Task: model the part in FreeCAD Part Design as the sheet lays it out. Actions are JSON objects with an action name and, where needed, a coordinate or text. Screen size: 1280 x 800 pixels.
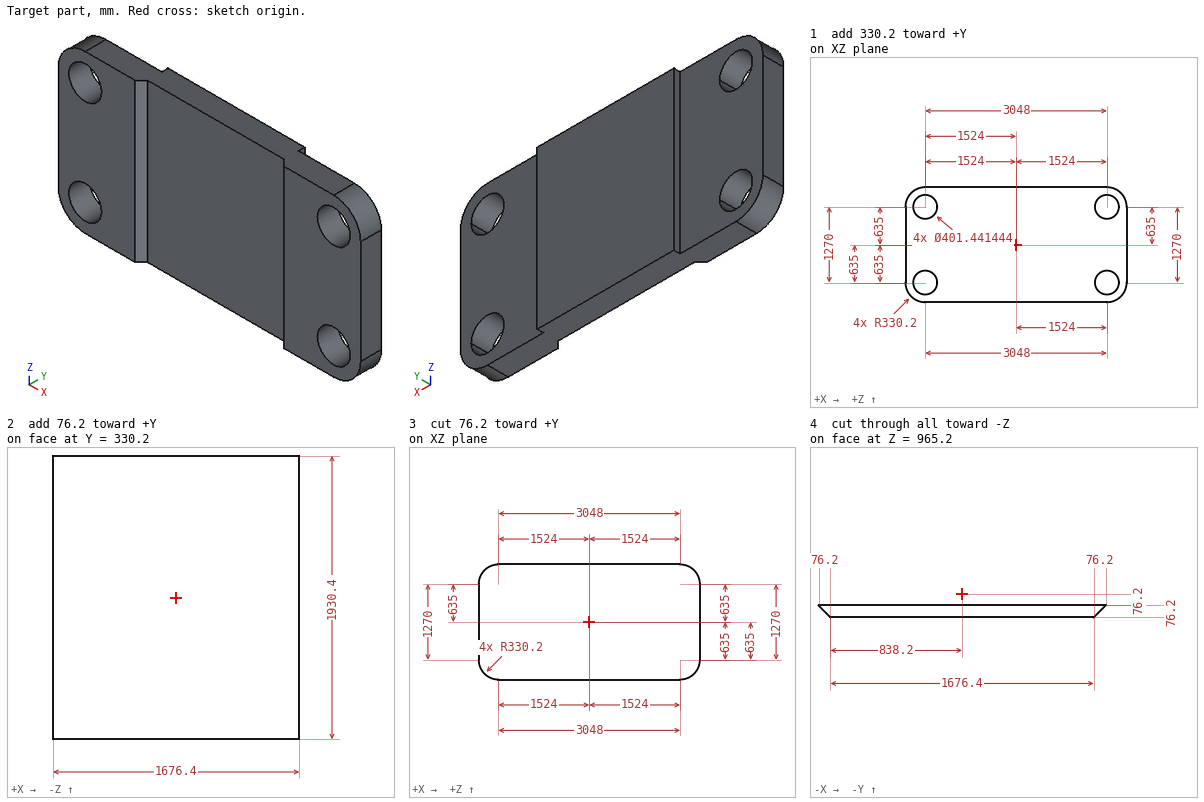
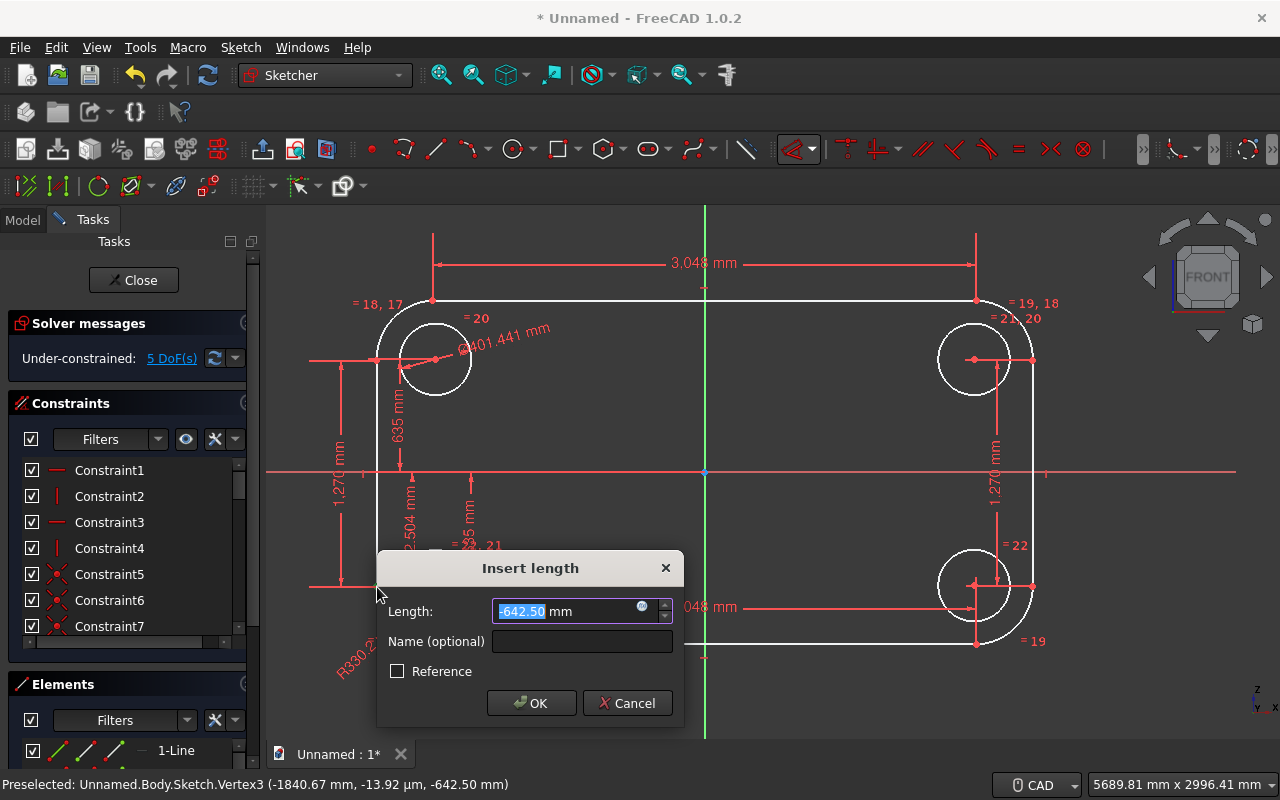
{"action": "type", "text": "-635"}
{"action": "key", "text": "Return"}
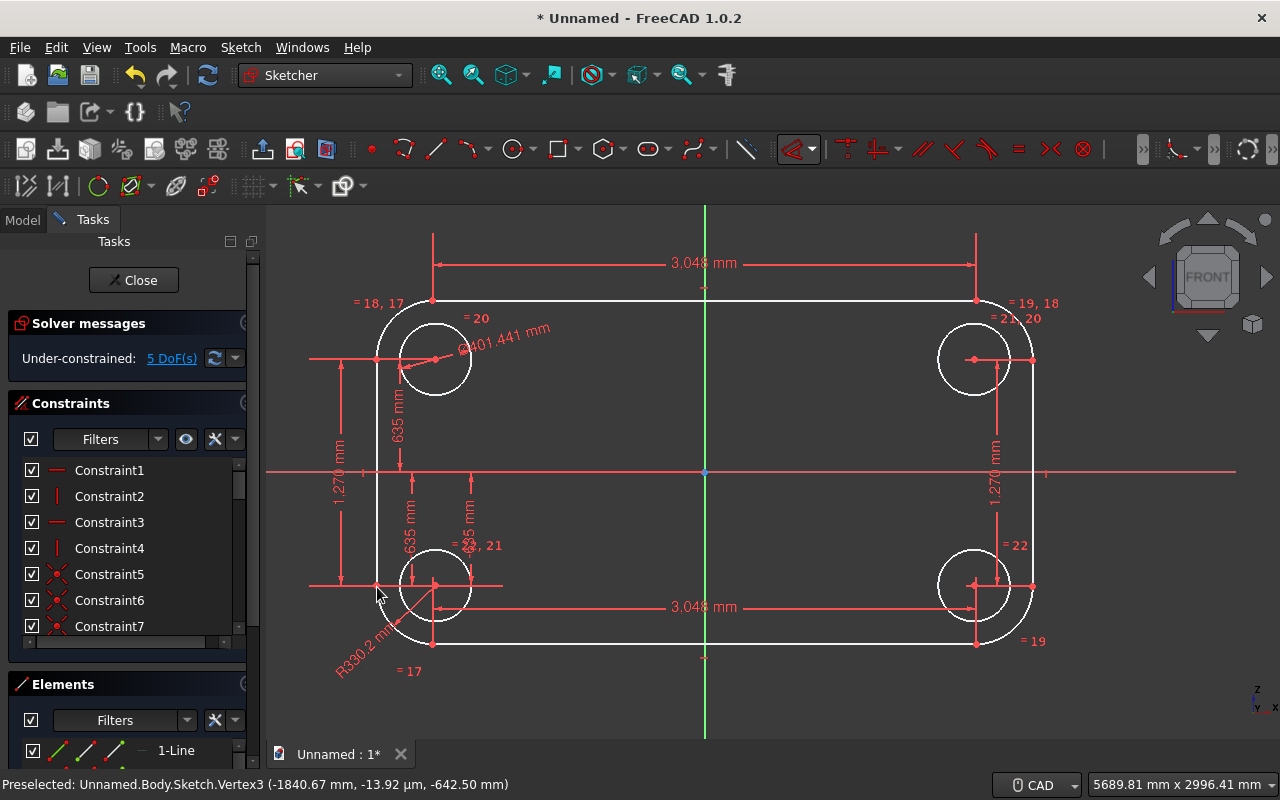
{"action": "left_click", "coordinate": [1033, 360]}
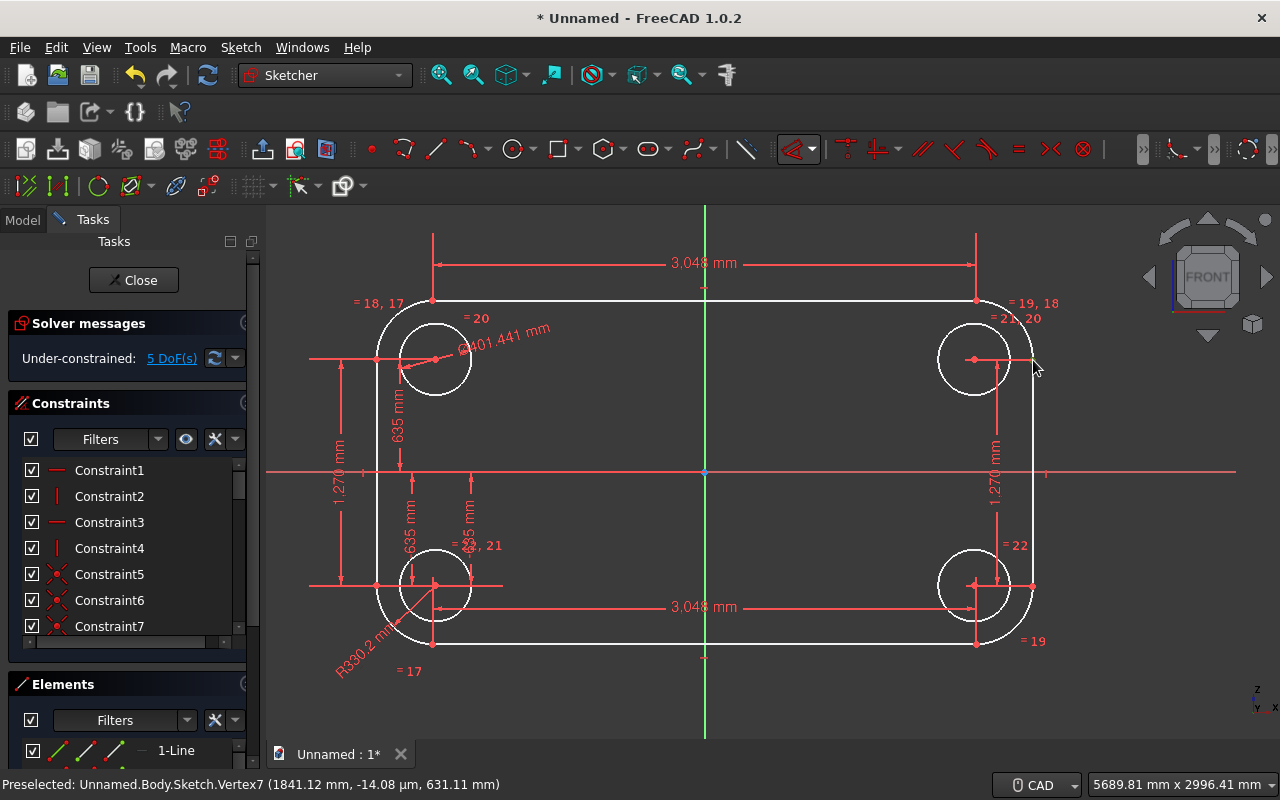
{"action": "left_click", "coordinate": [814, 150]}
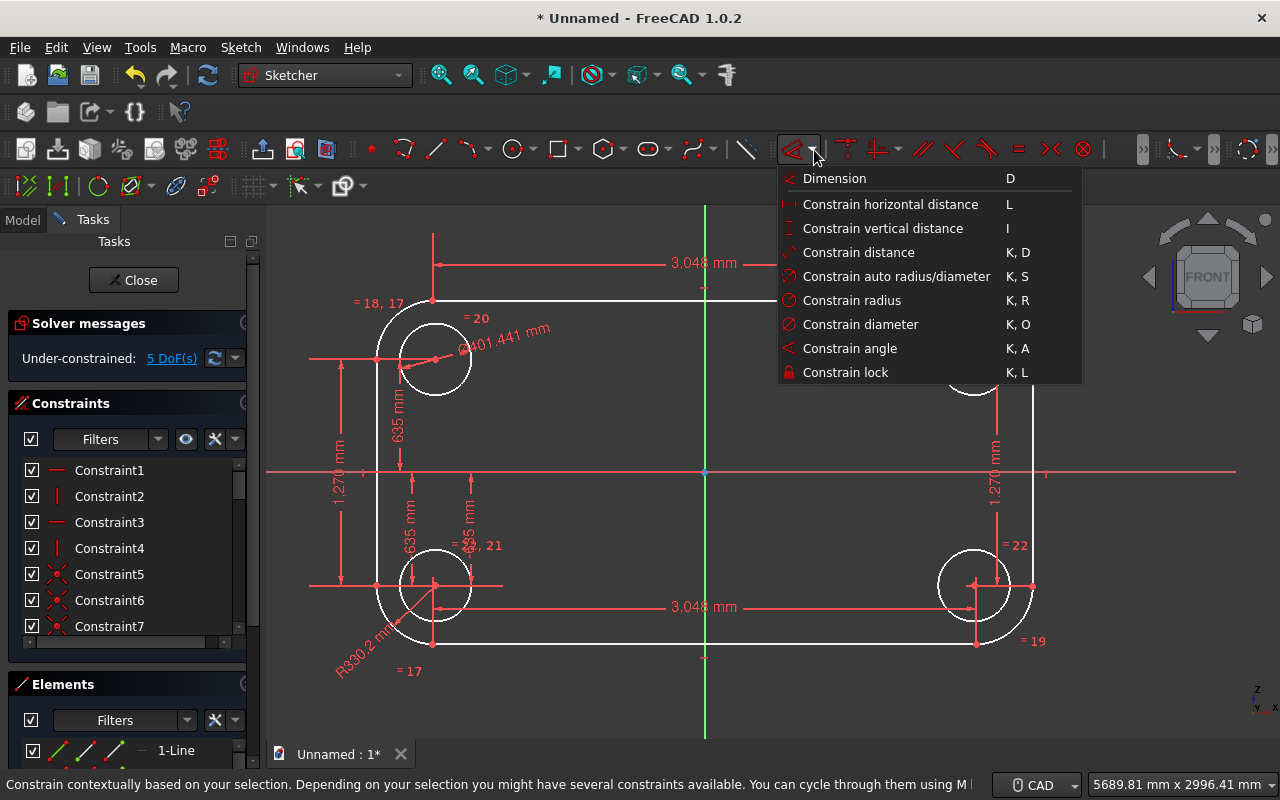
{"action": "left_click", "coordinate": [930, 228]}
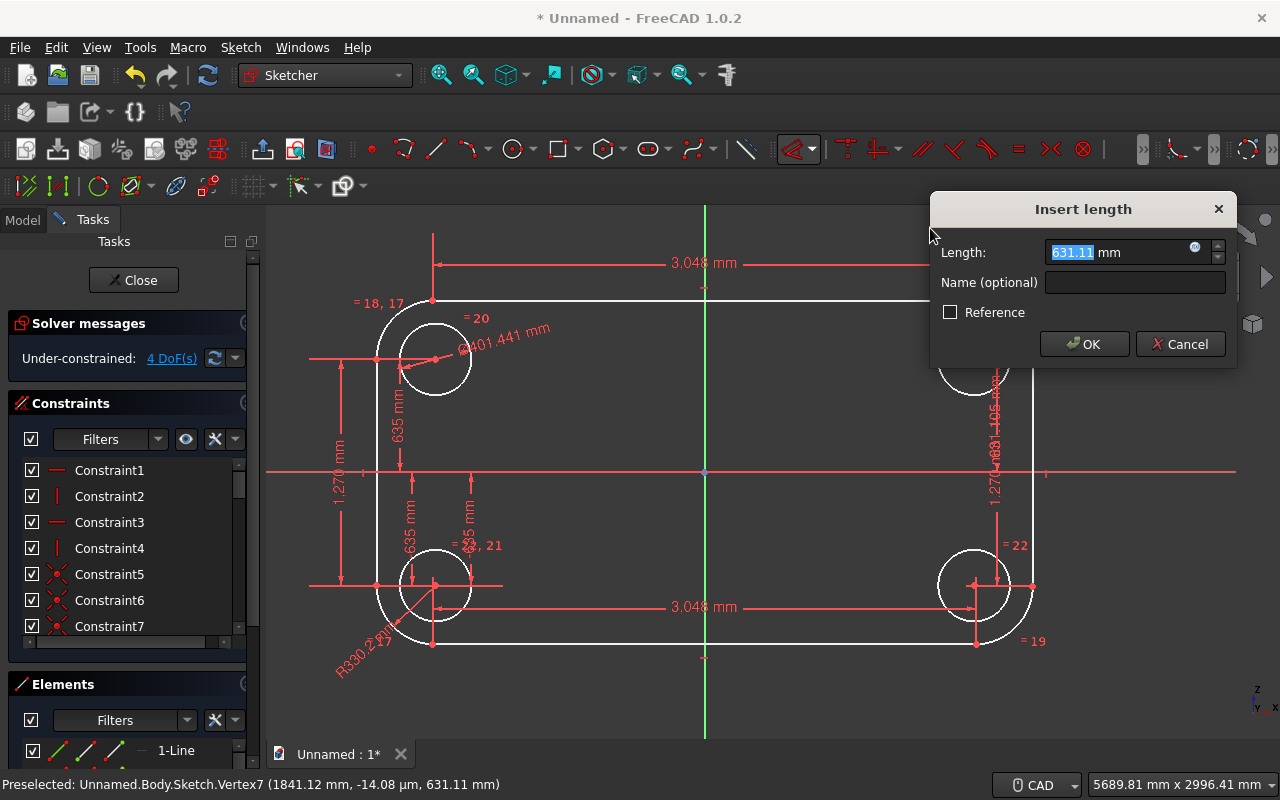
{"action": "type", "text": "635"}
{"action": "key", "text": "Return"}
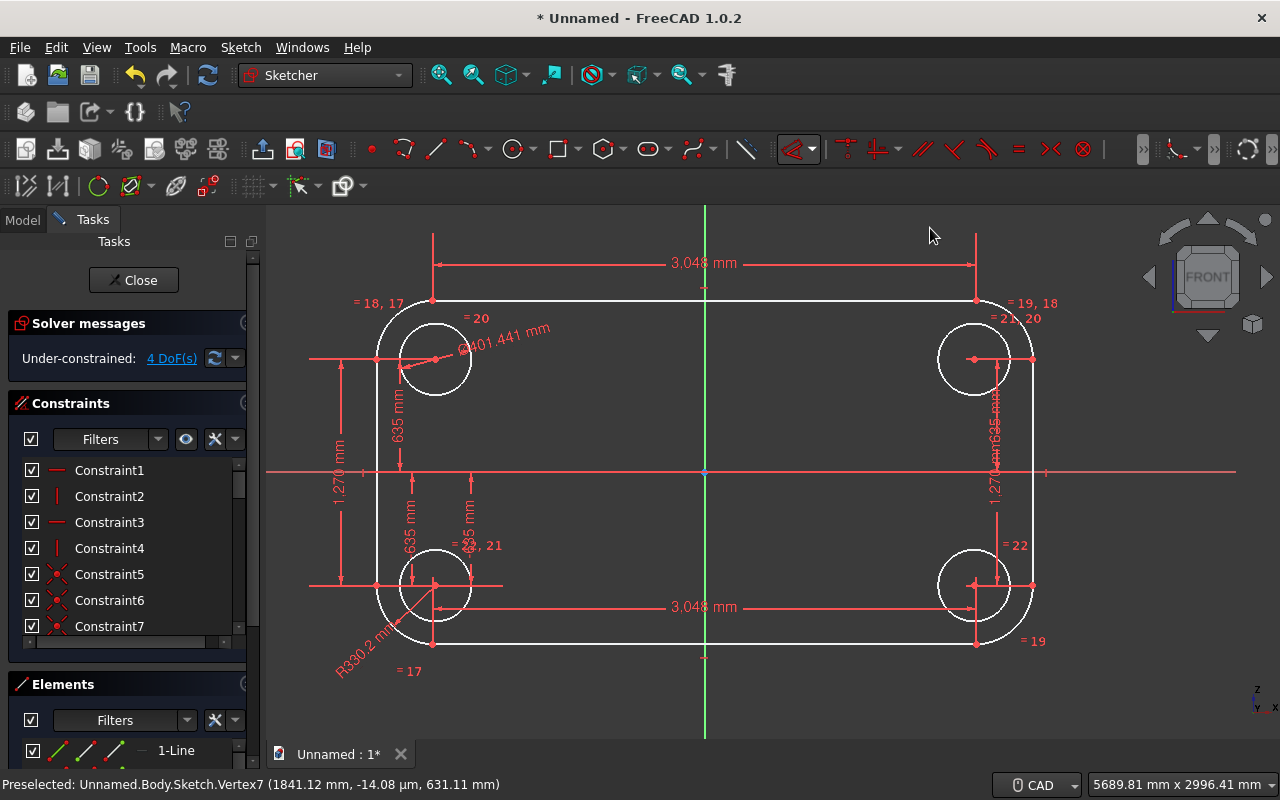
{"action": "left_click", "coordinate": [436, 359]}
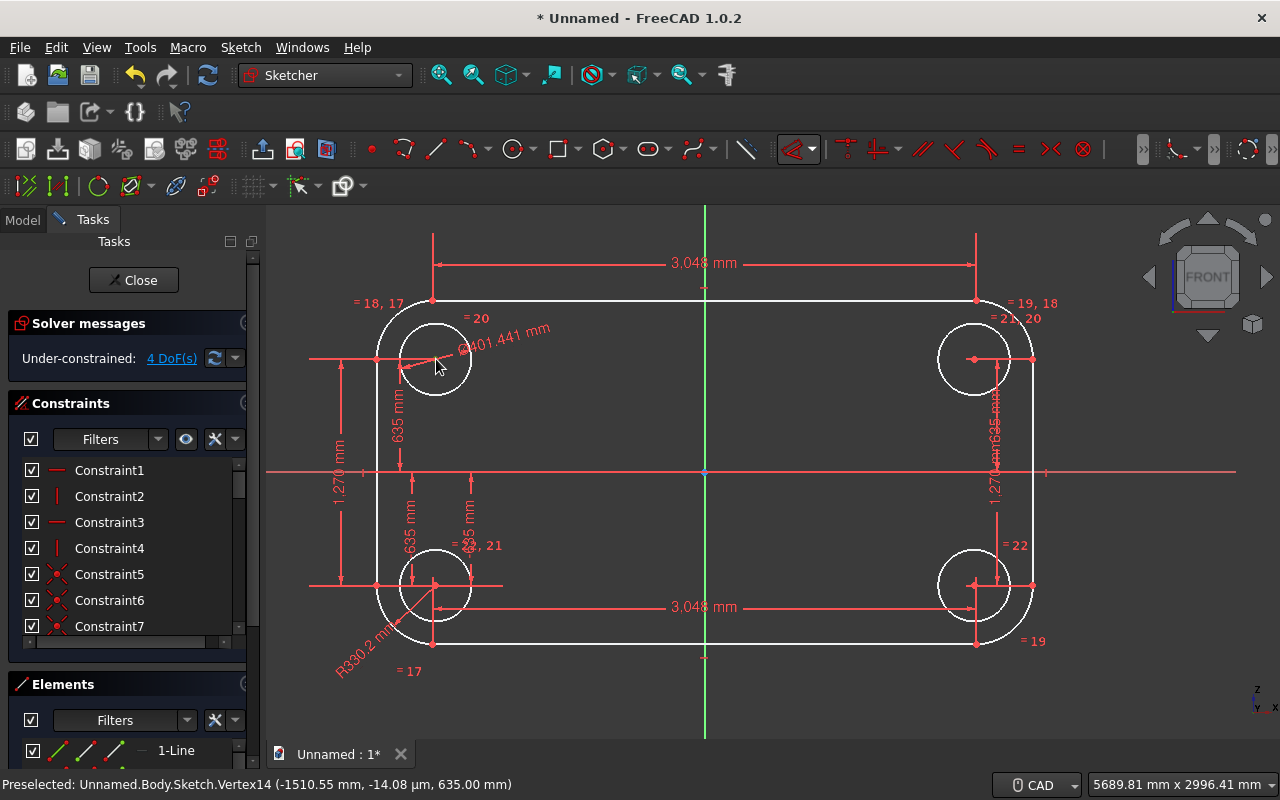
{"action": "key", "text": "l"}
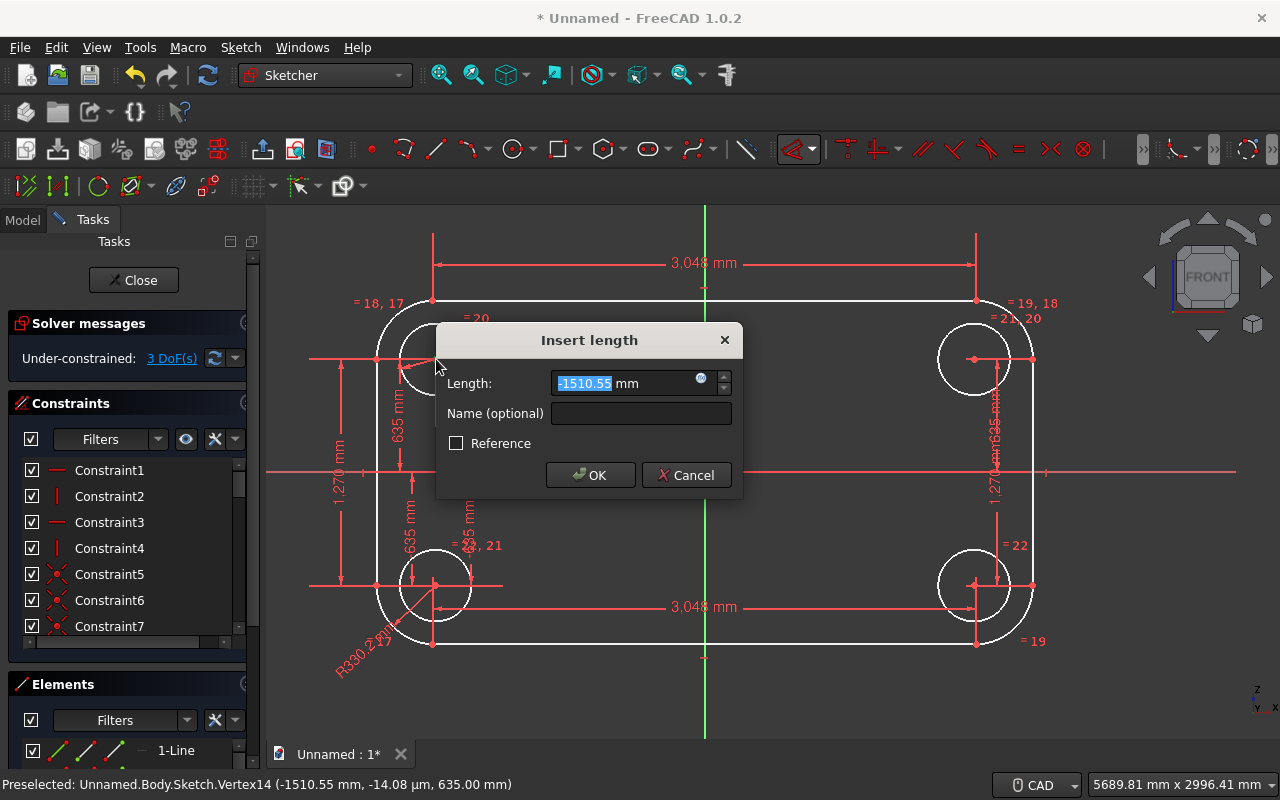
{"action": "type", "text": "-1524"}
{"action": "key", "text": "Return"}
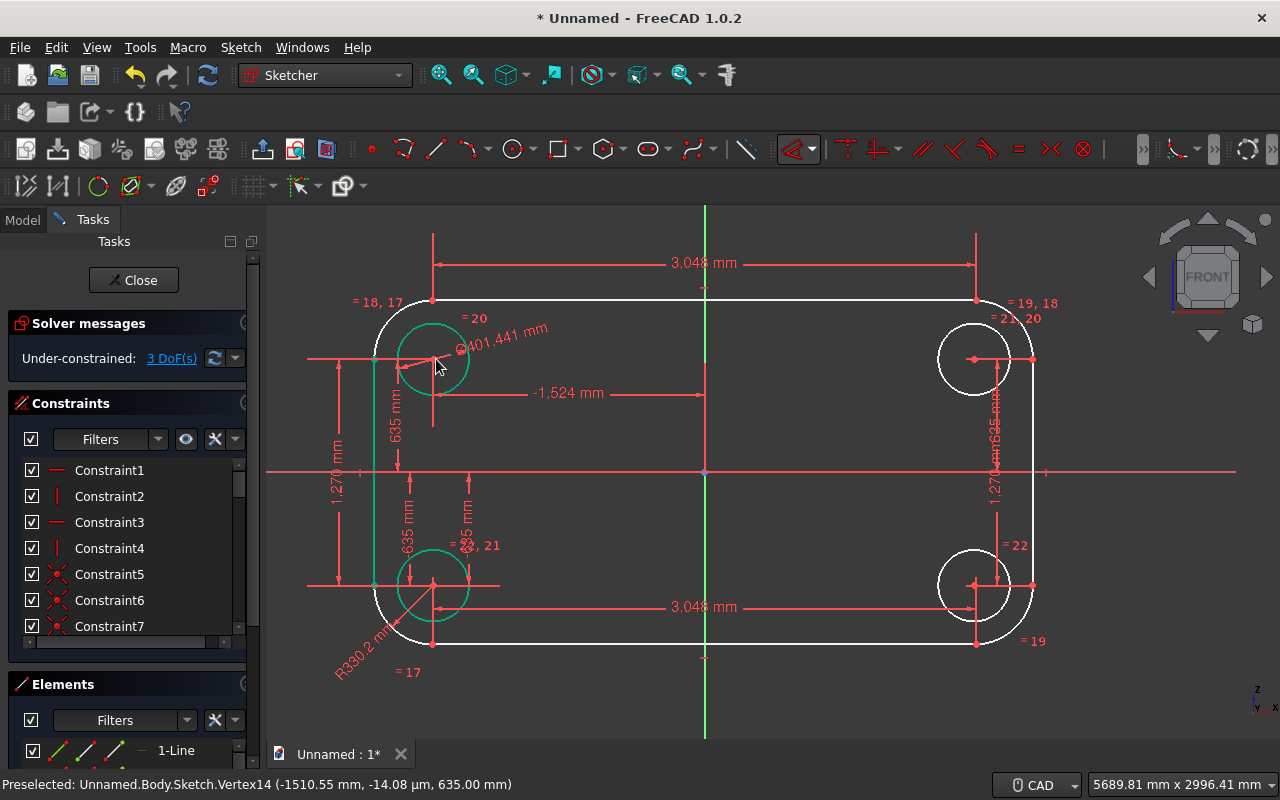
{"action": "left_click", "coordinate": [974, 359]}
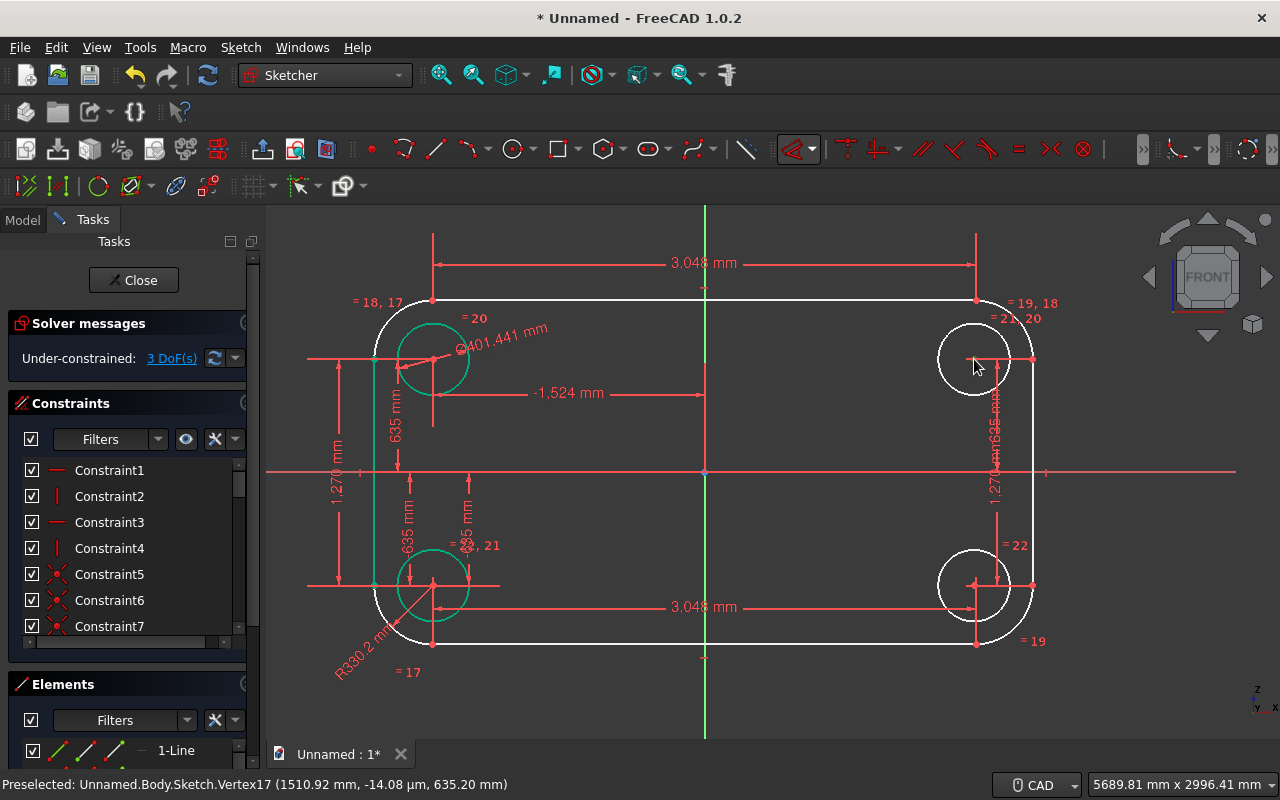
{"action": "key", "text": "l"}